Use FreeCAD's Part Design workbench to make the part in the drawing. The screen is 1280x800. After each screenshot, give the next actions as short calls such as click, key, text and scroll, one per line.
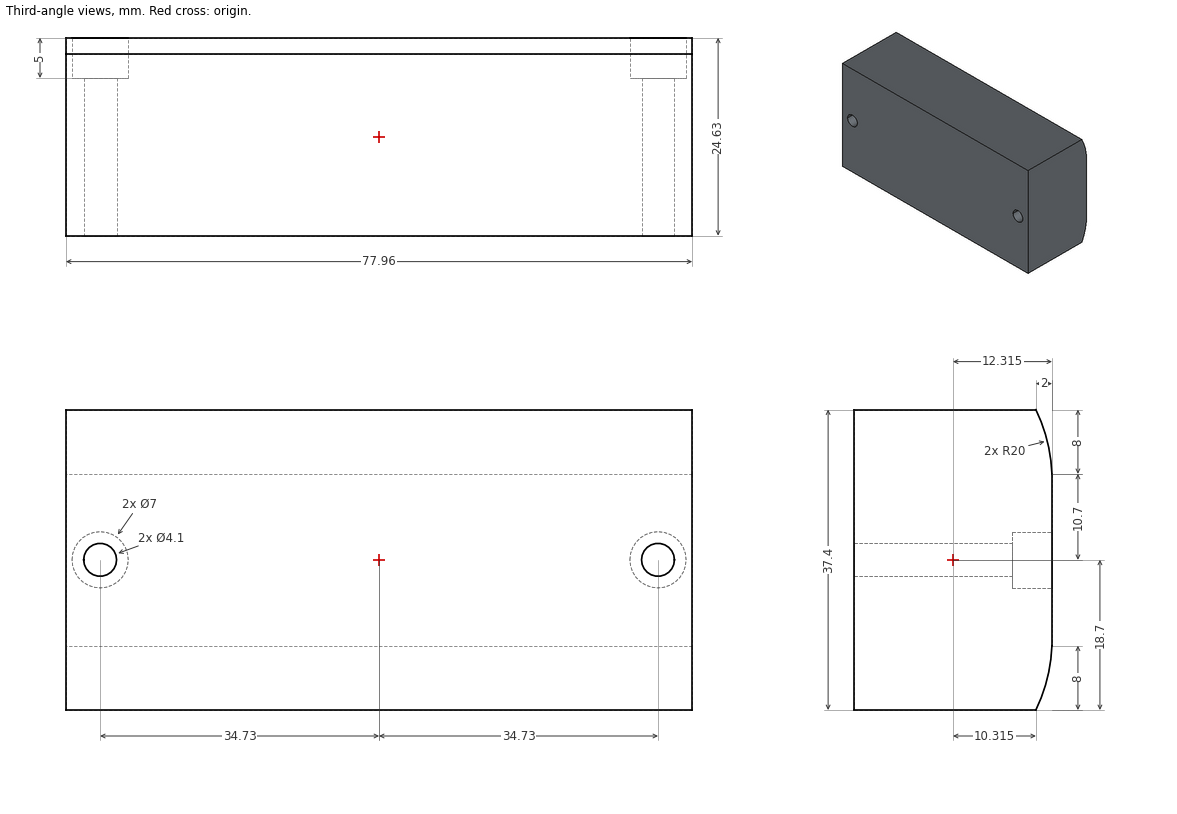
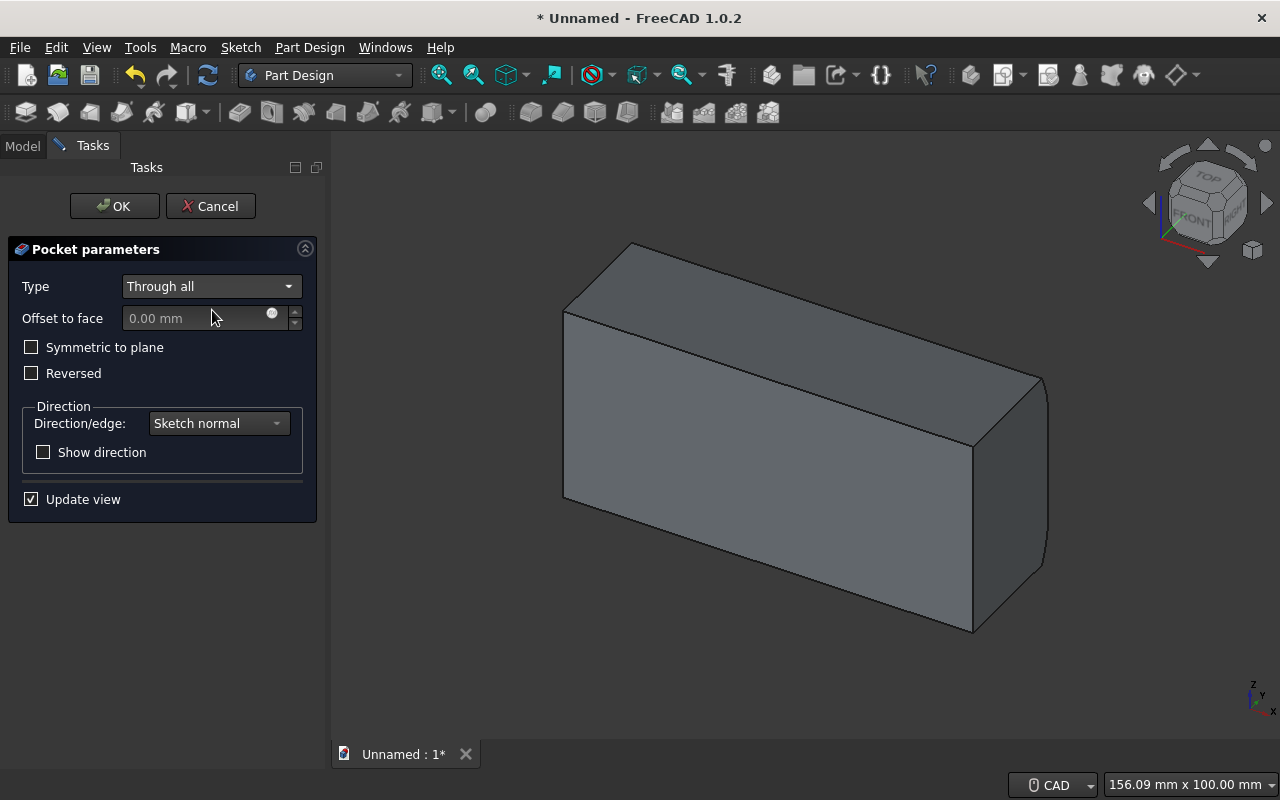
click(115, 206)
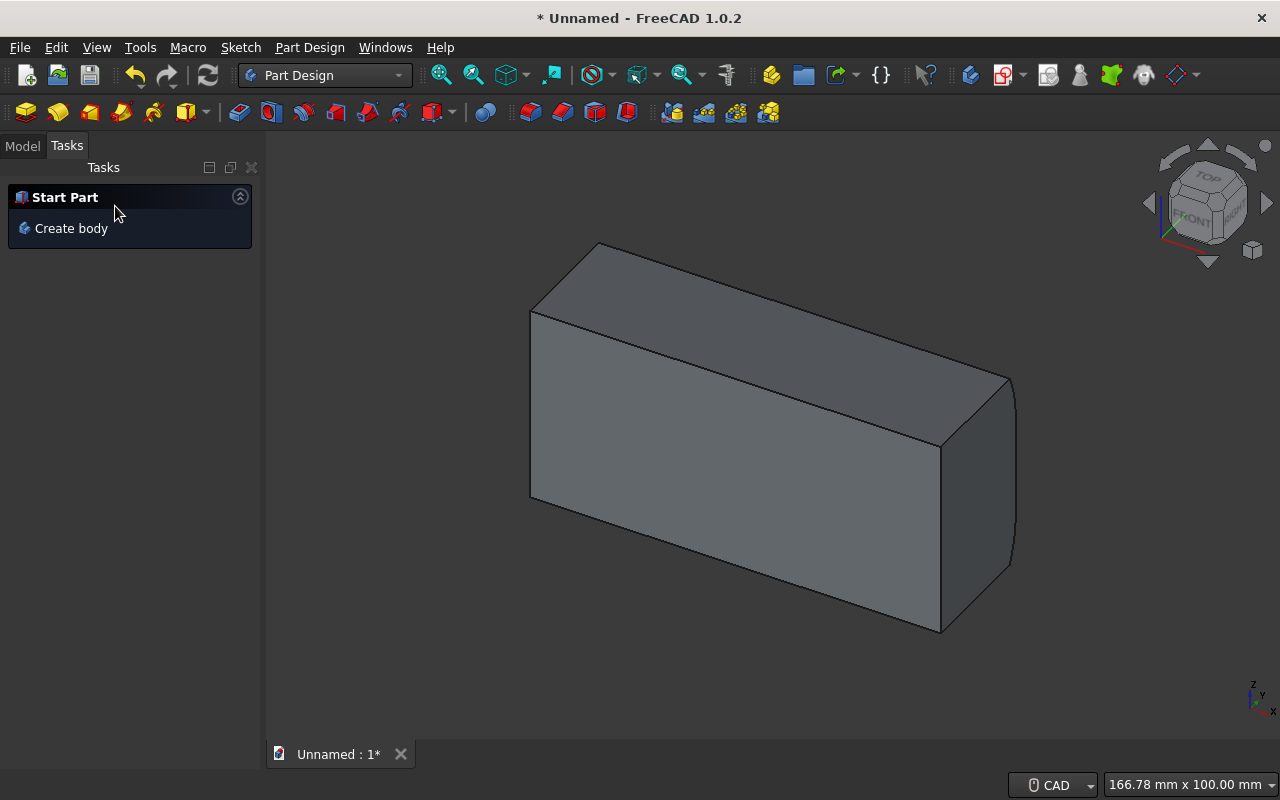
key(4)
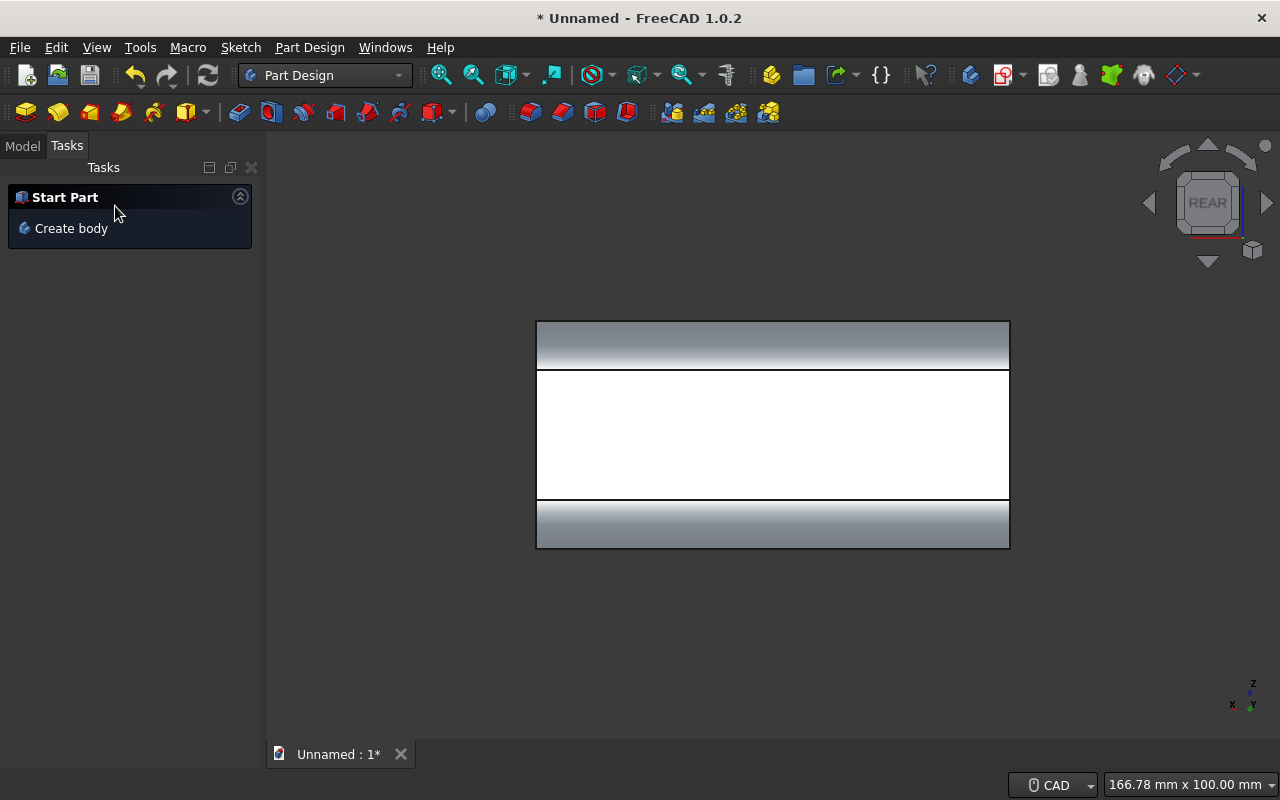
click(638, 434)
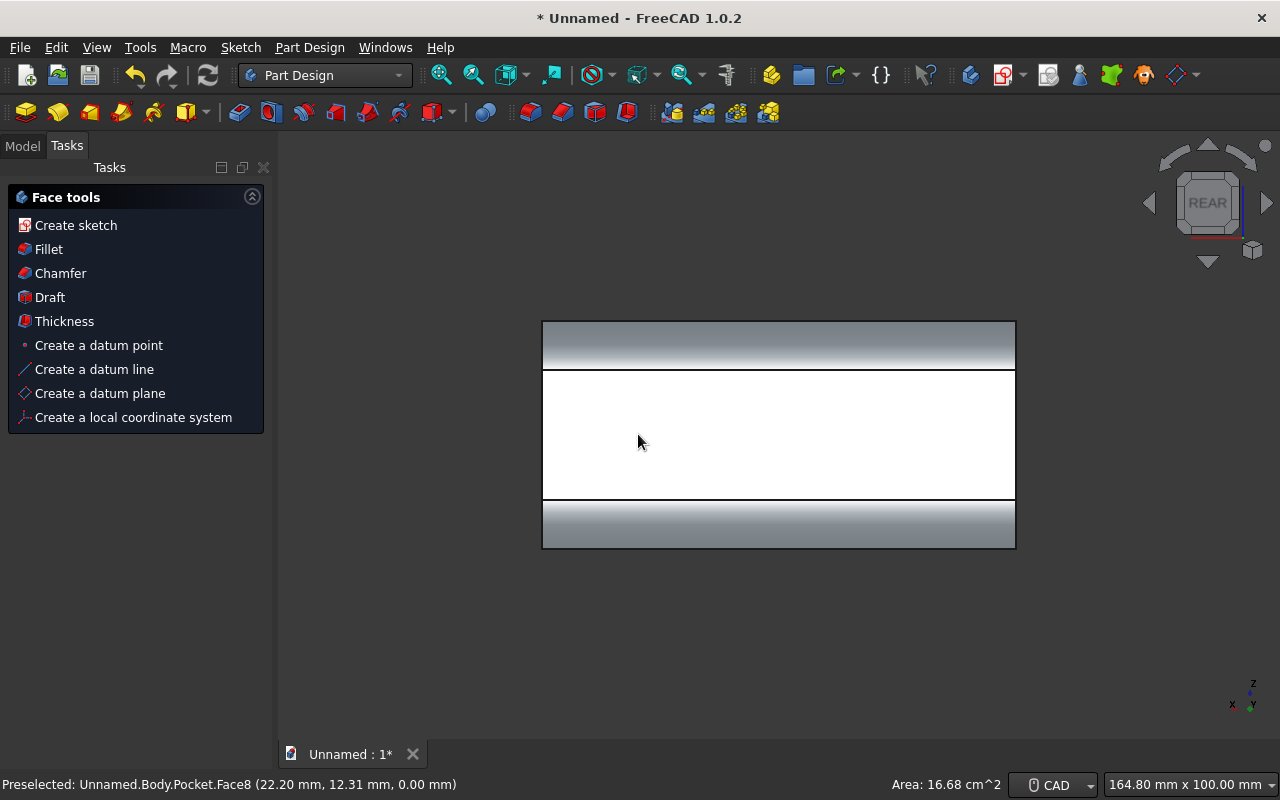
click(1004, 76)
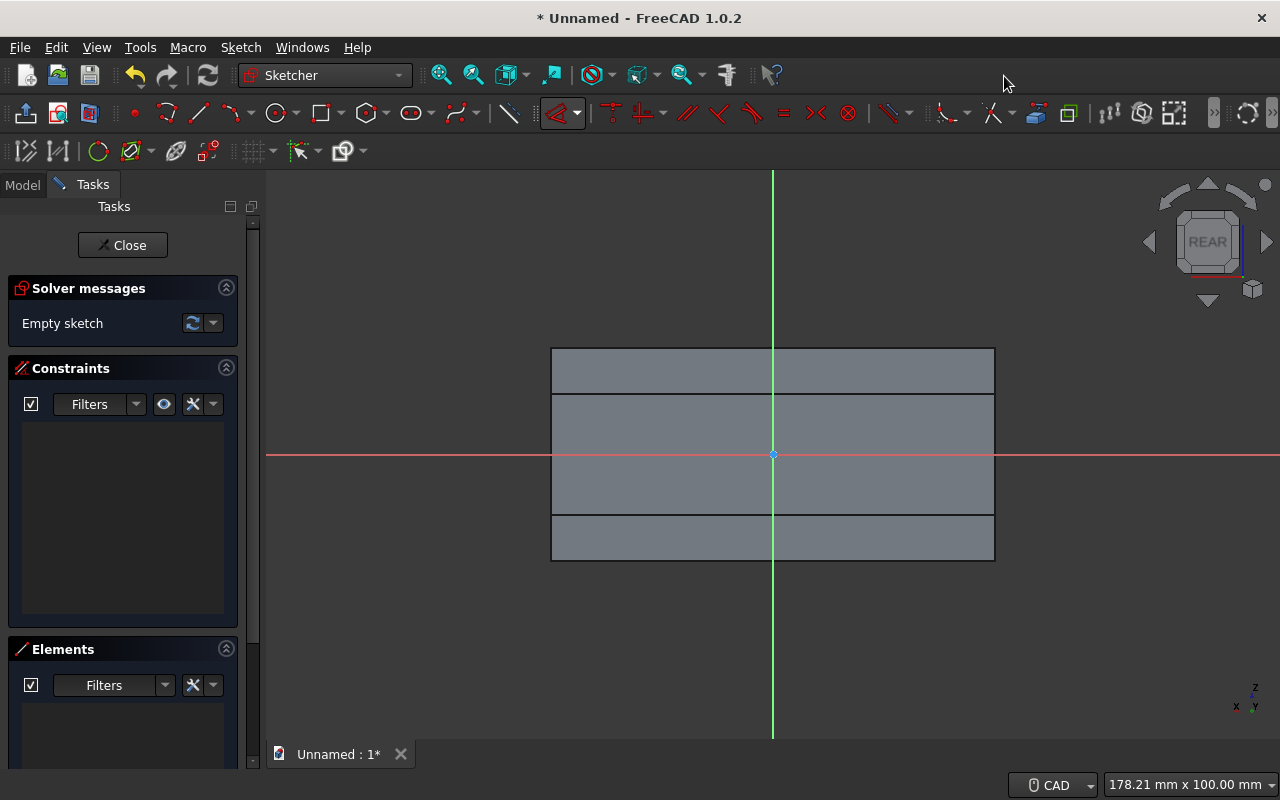
scroll(912, 454, up, 2)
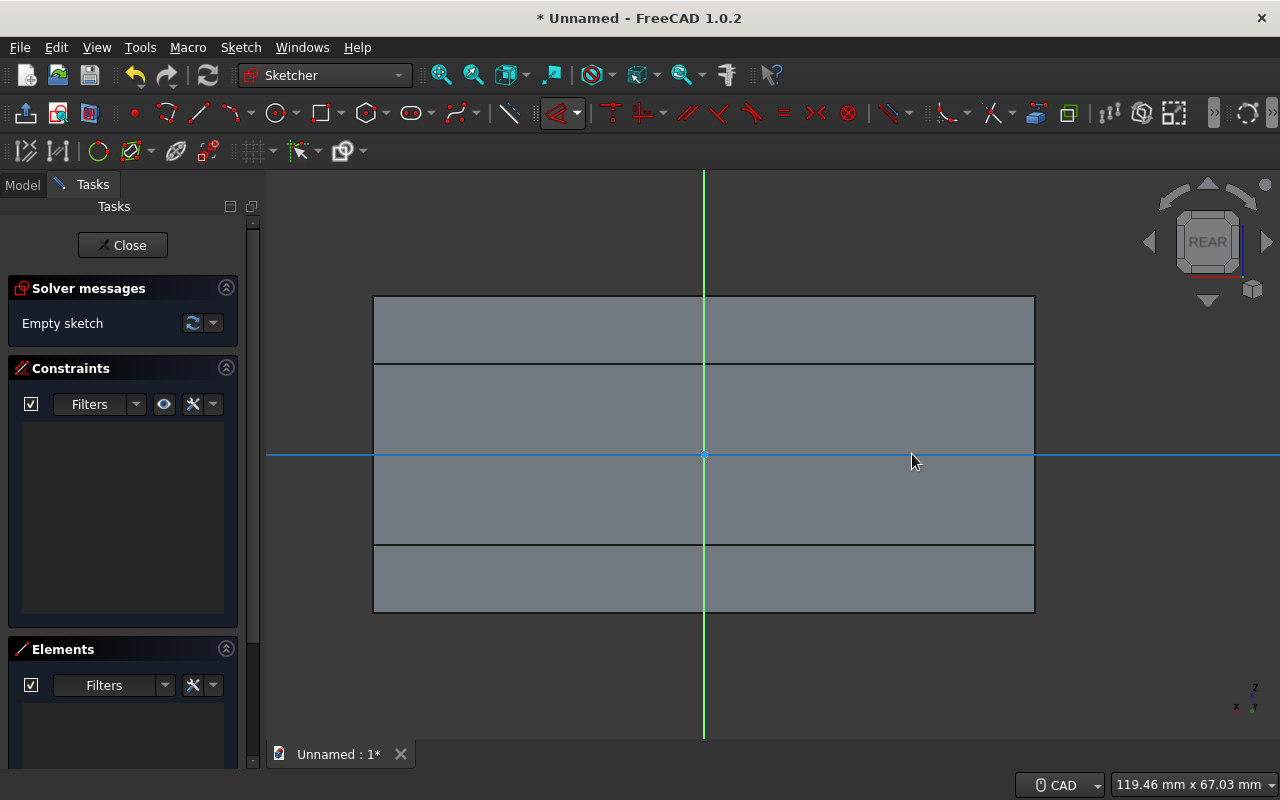
click(276, 114)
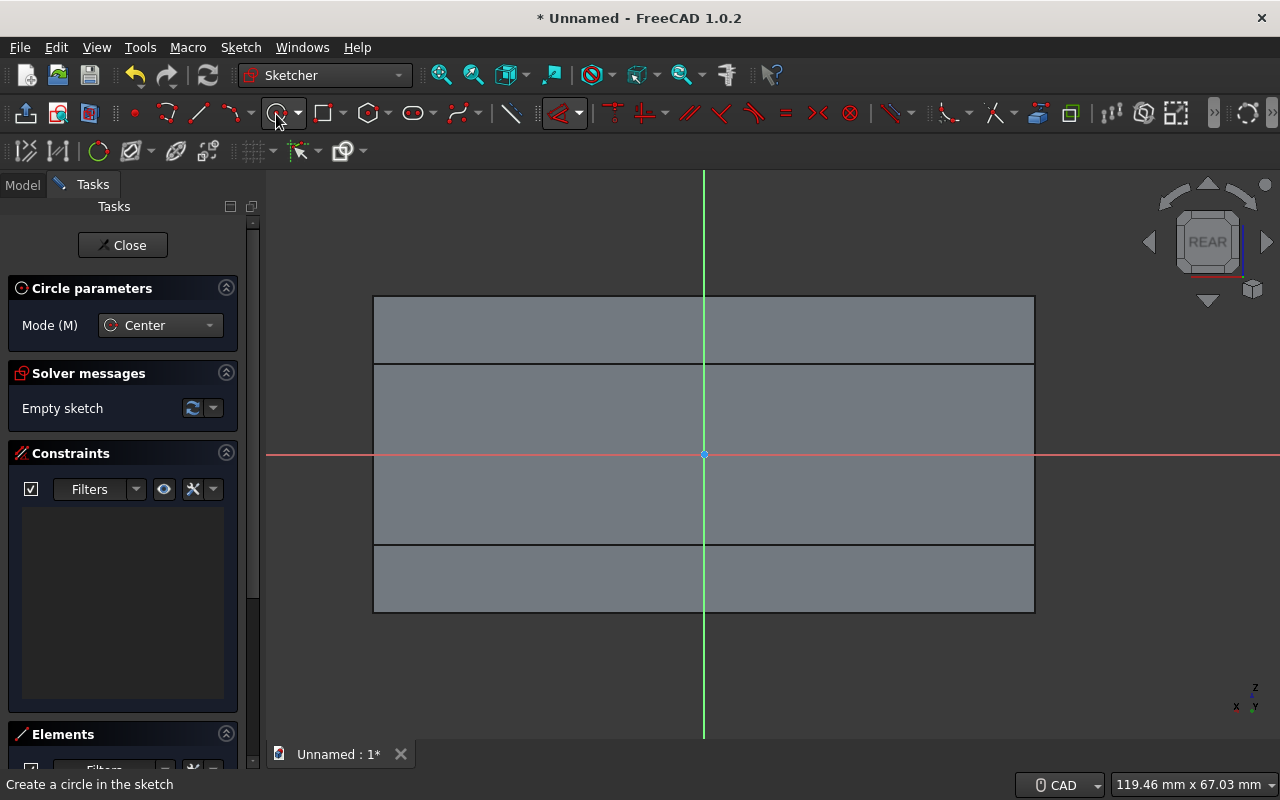
scroll(999, 454, up, 2)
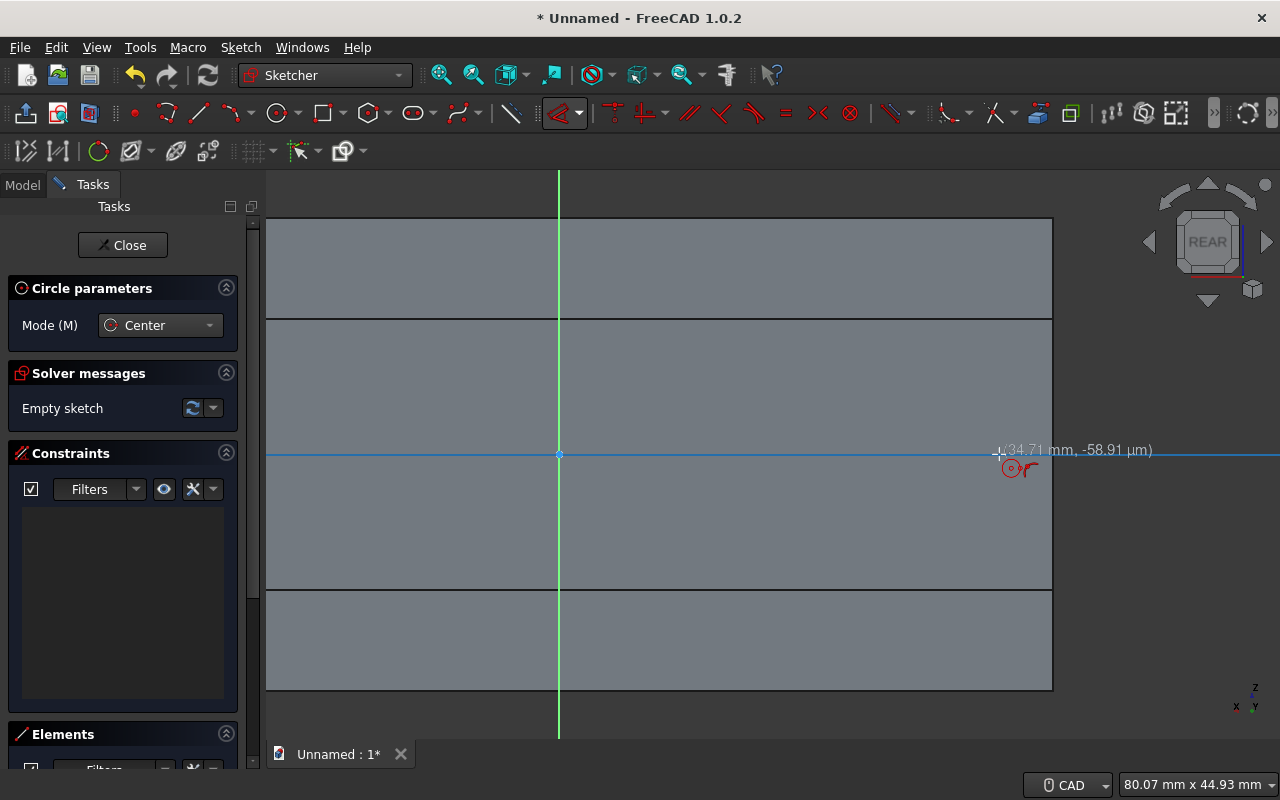
click(999, 454)
click(1017, 436)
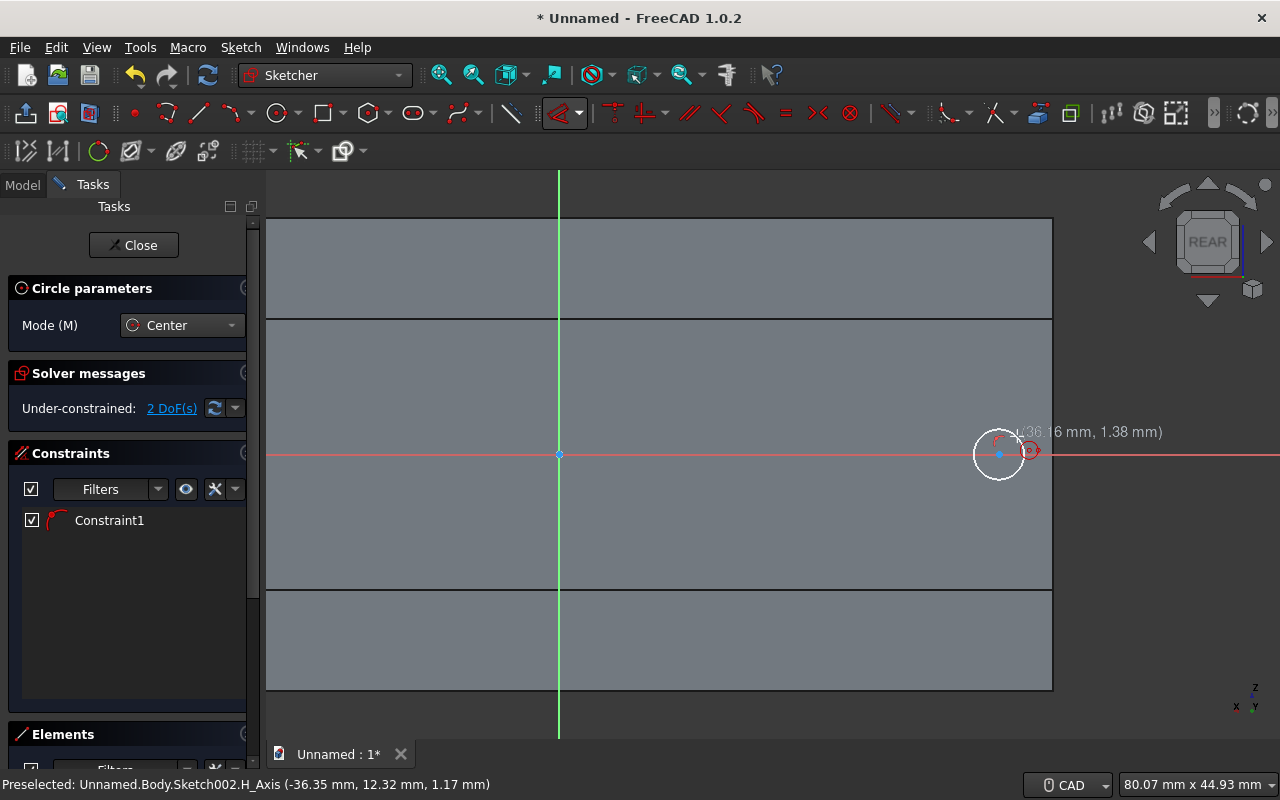
scroll(1000, 455, down, 2)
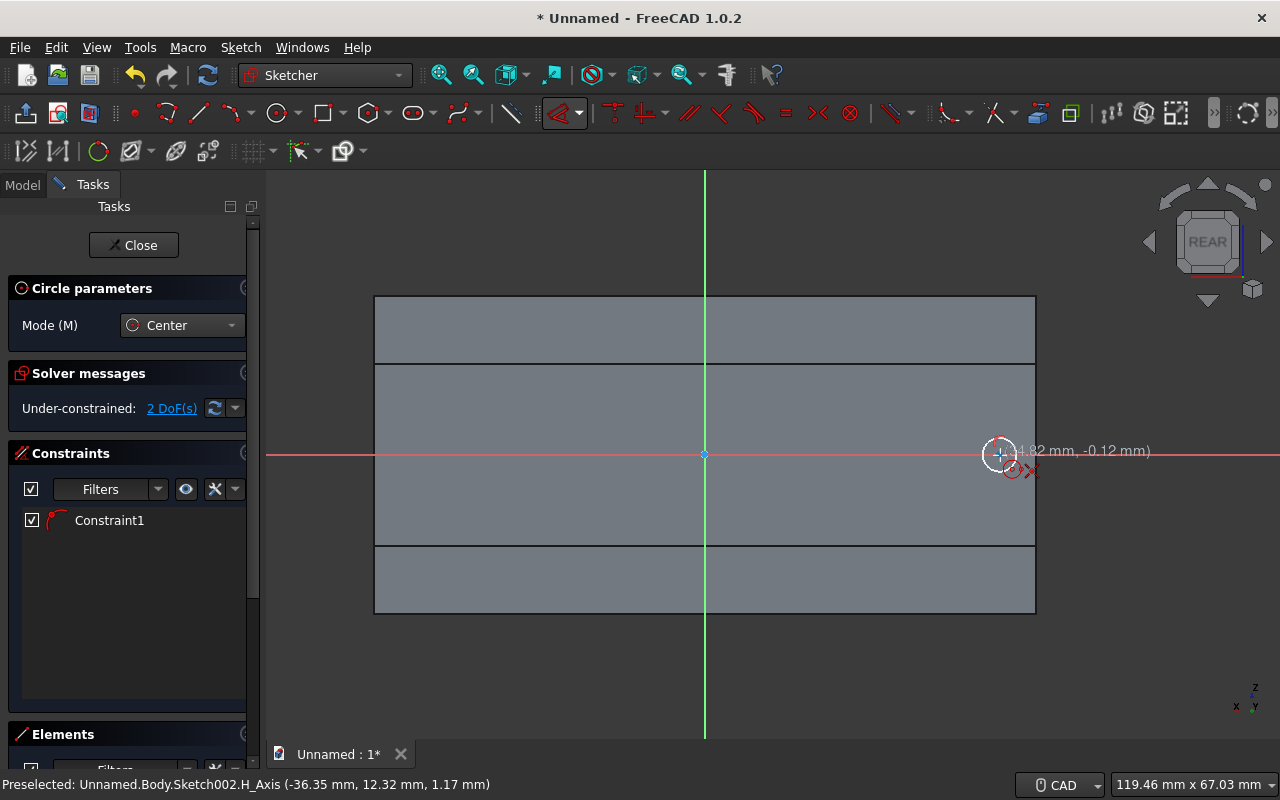
scroll(410, 455, up, 2)